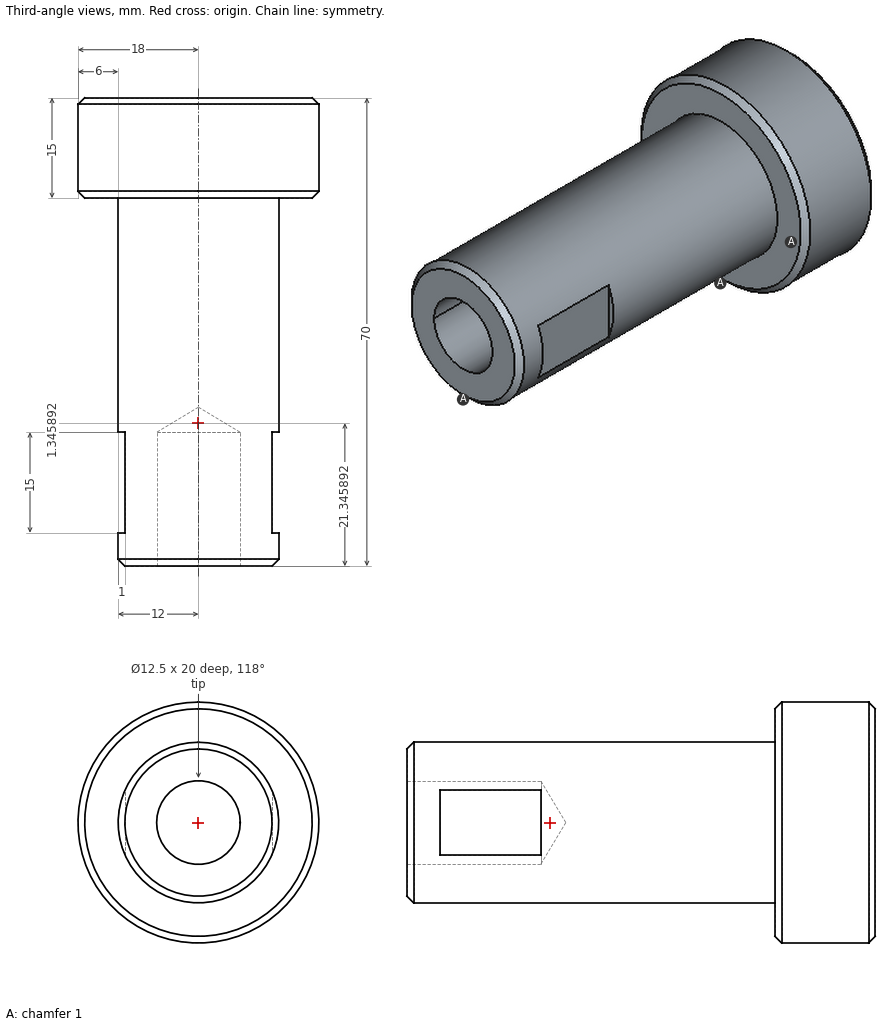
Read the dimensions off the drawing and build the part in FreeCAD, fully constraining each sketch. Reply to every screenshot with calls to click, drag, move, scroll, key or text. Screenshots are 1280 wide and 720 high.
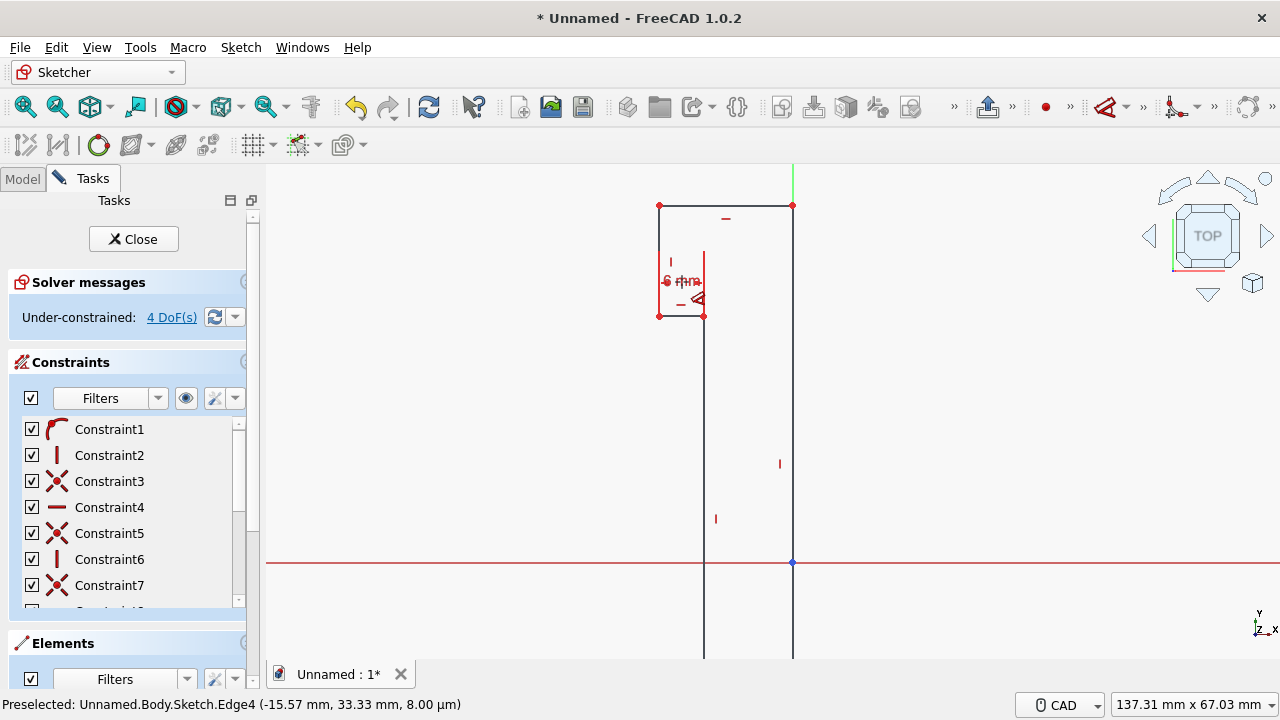
click(793, 567)
click(827, 418)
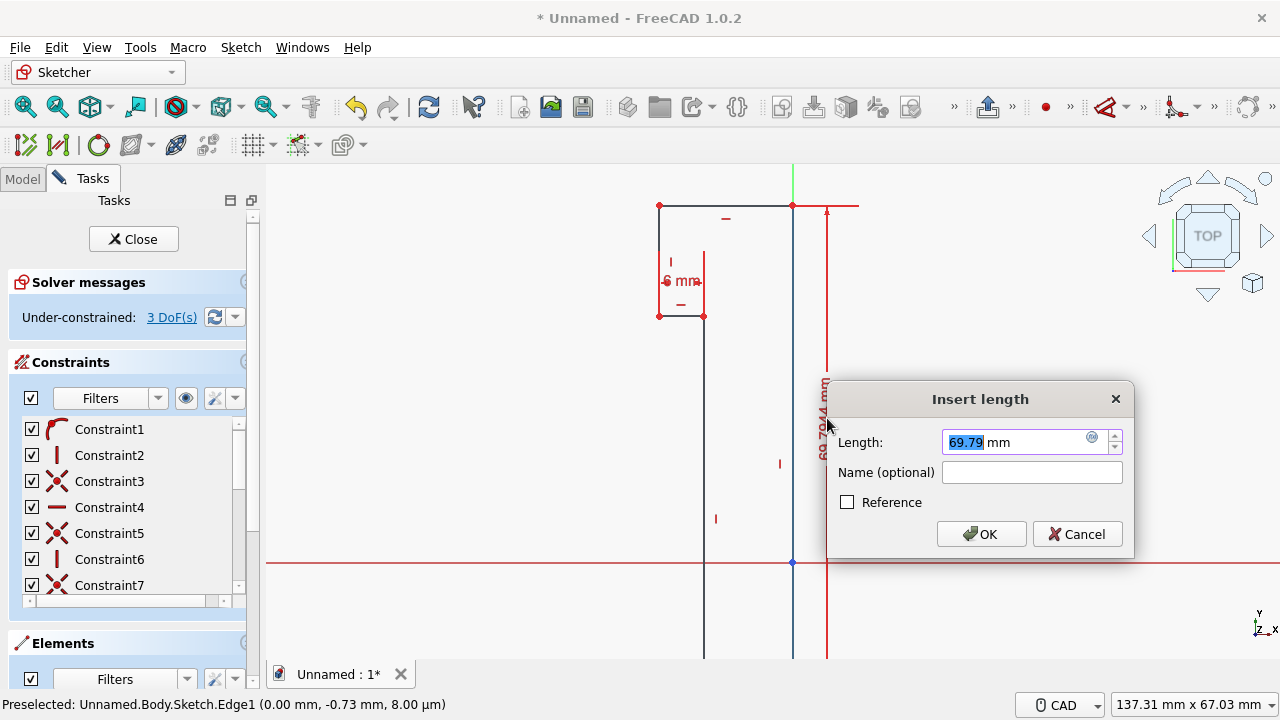
text(70)
key(Return)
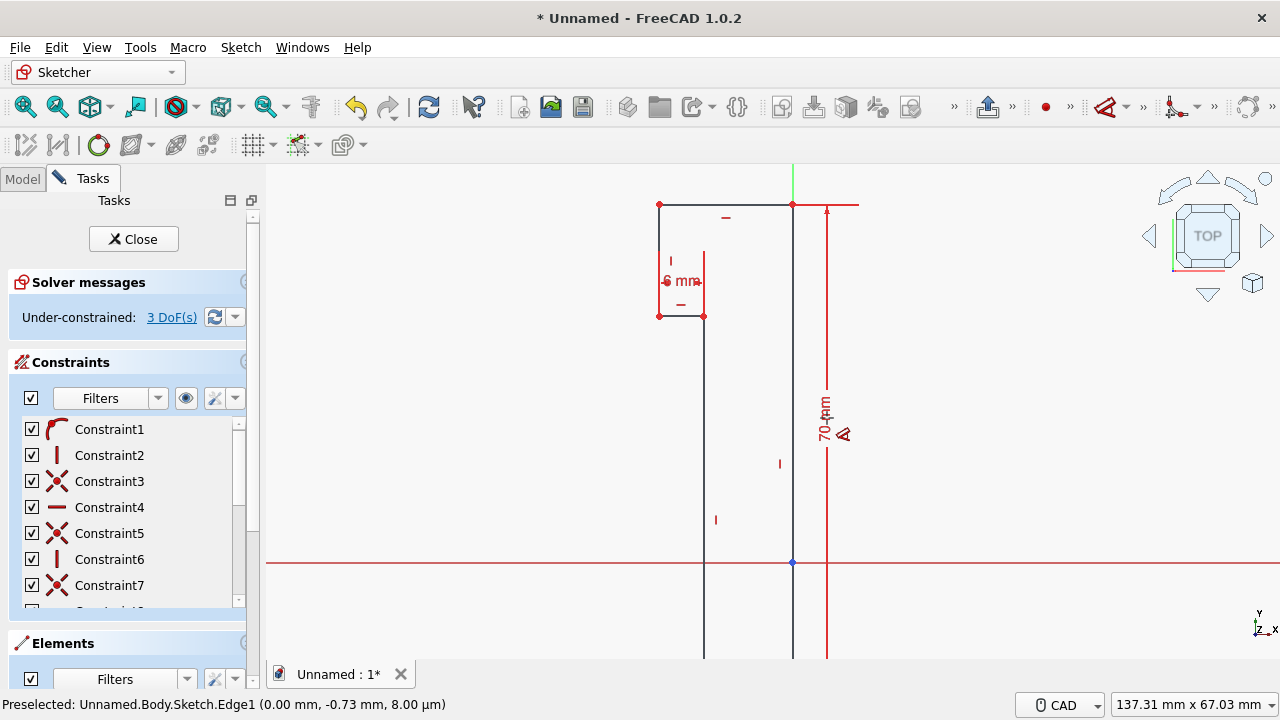
click(753, 205)
click(726, 239)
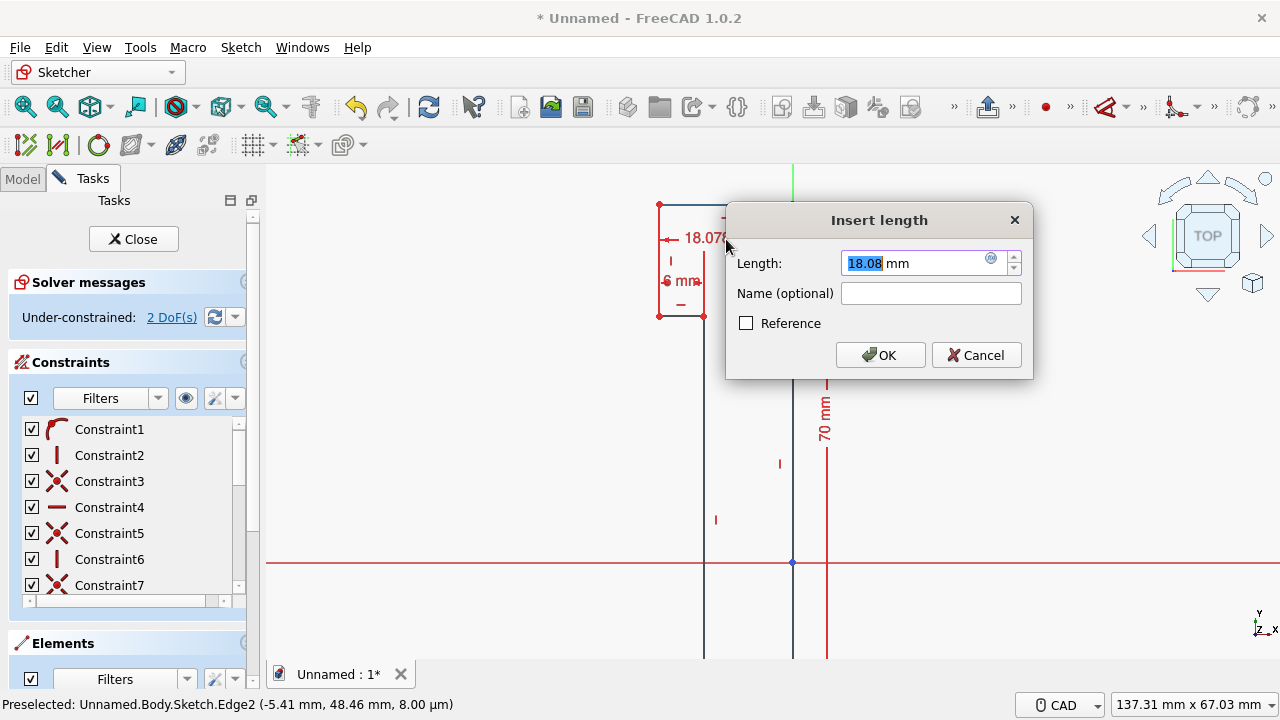
text(18)
key(Return)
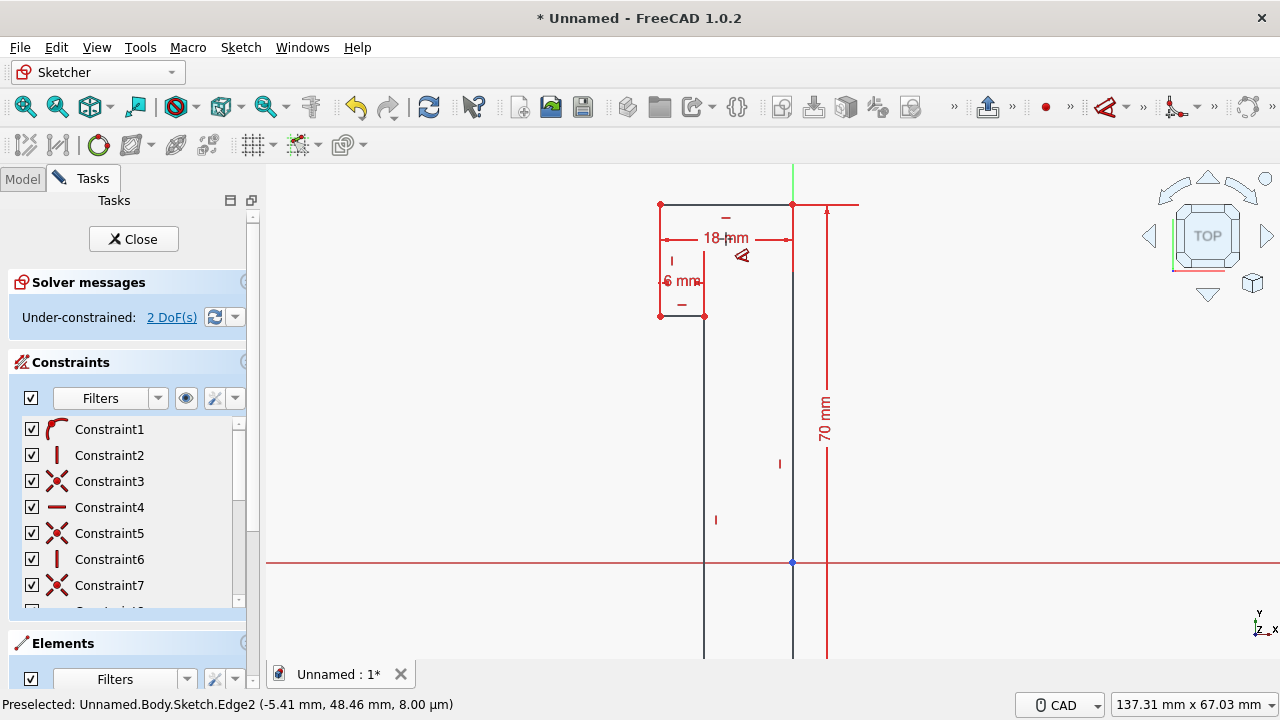
click(660, 238)
click(626, 261)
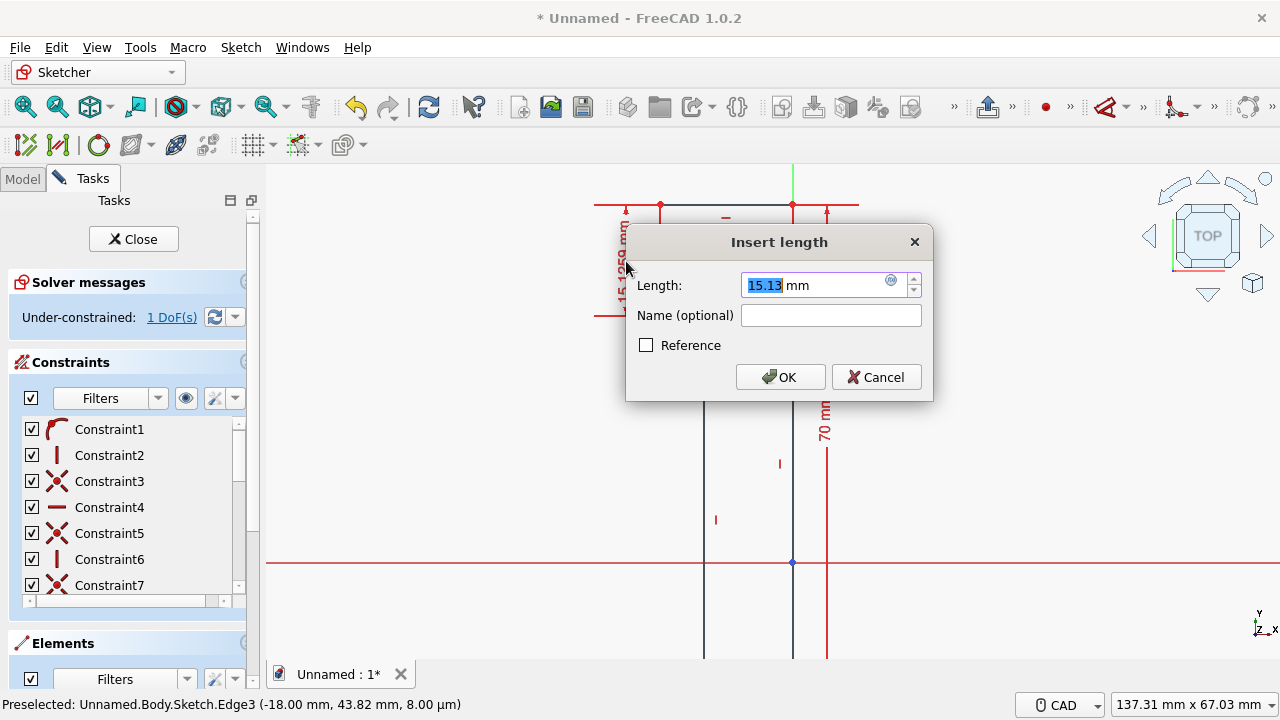
text(15)
key(Return)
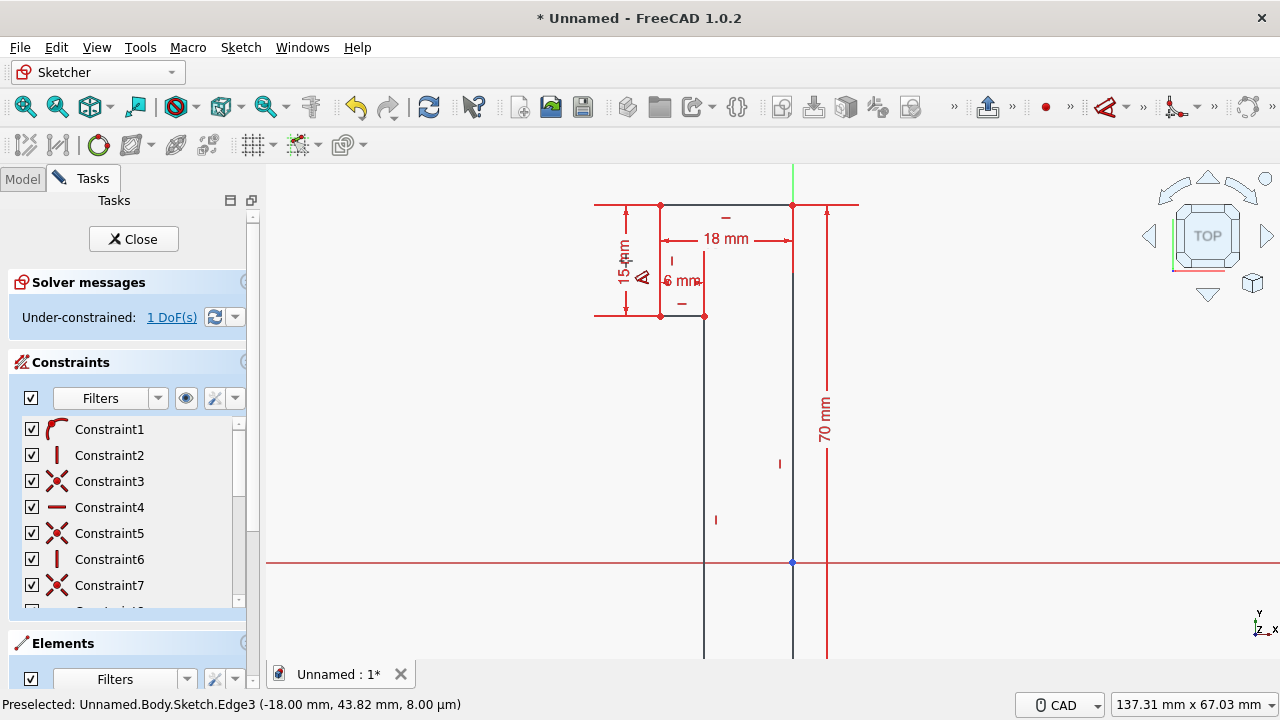
scroll(678, 350, down, 3)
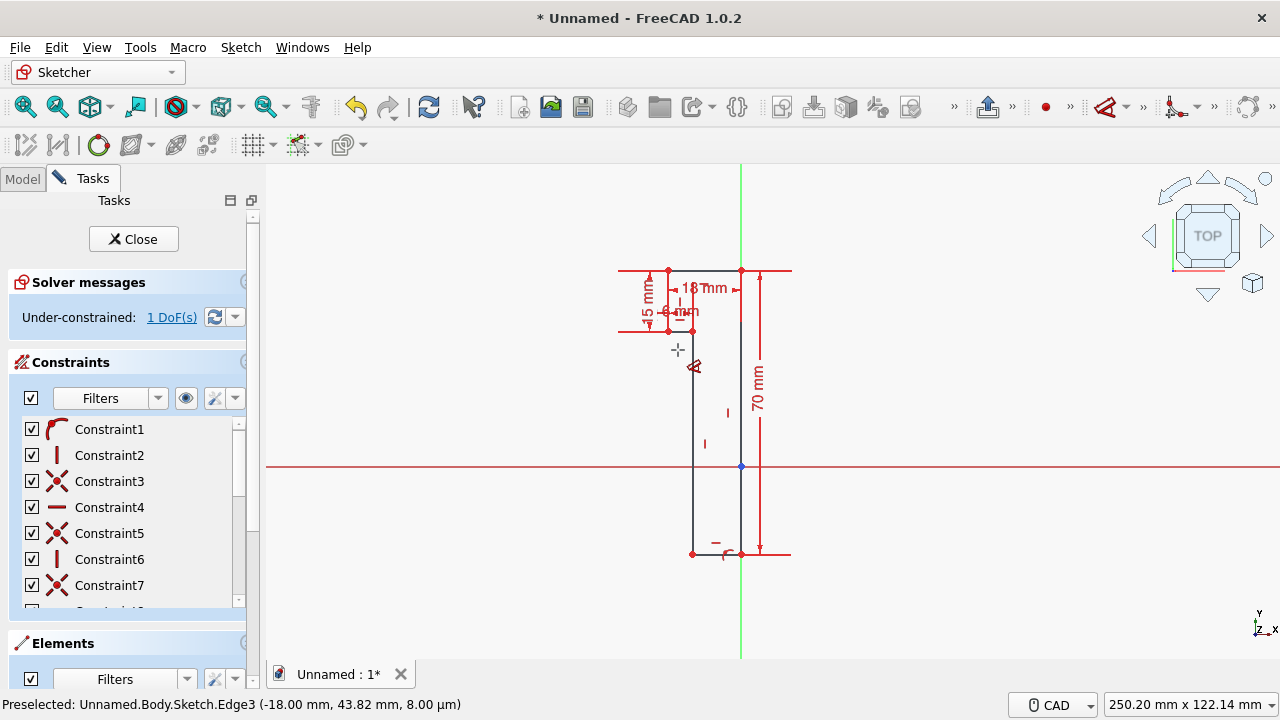
click(741, 555)
click(775, 511)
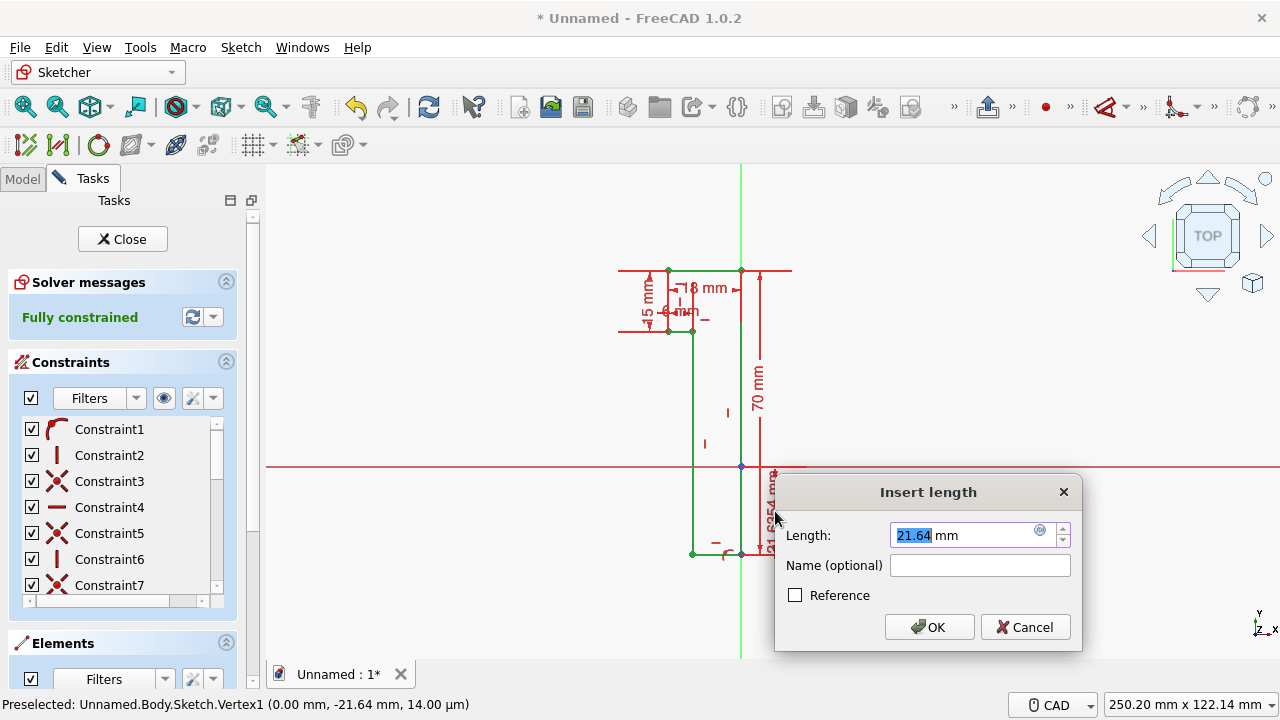
text(21.345892)
key(Return)
key(Escape)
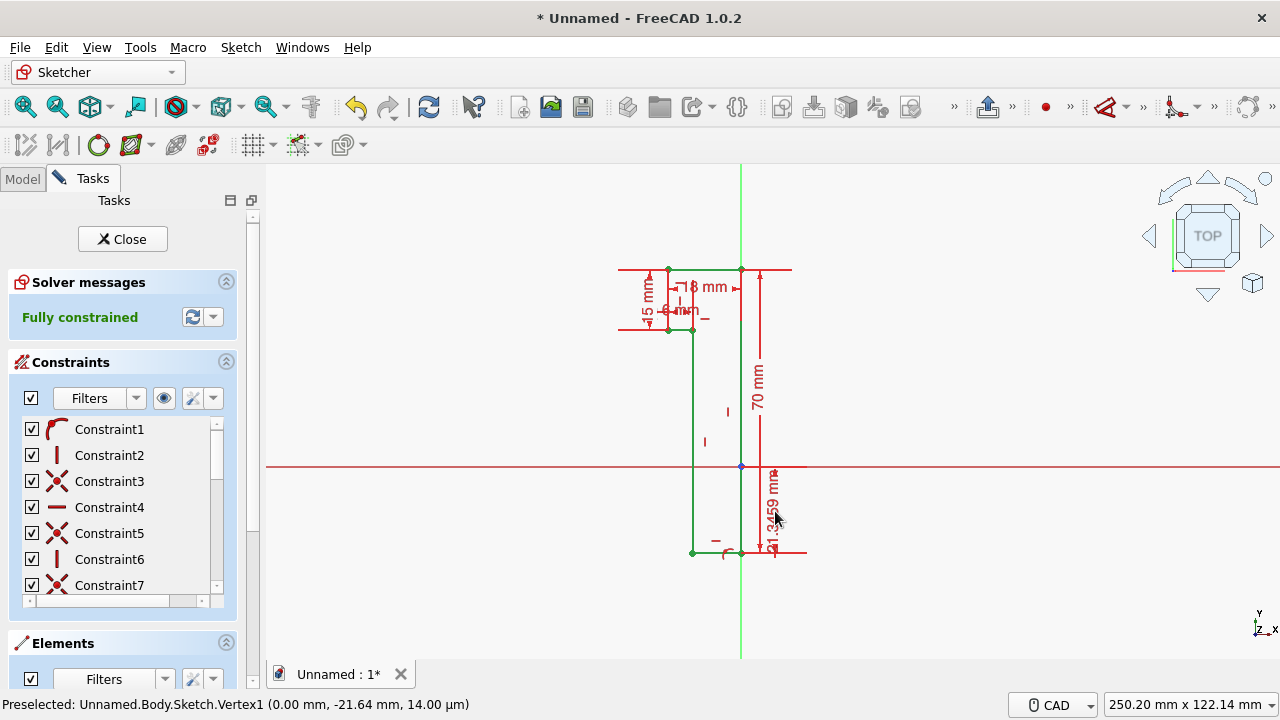
click(123, 239)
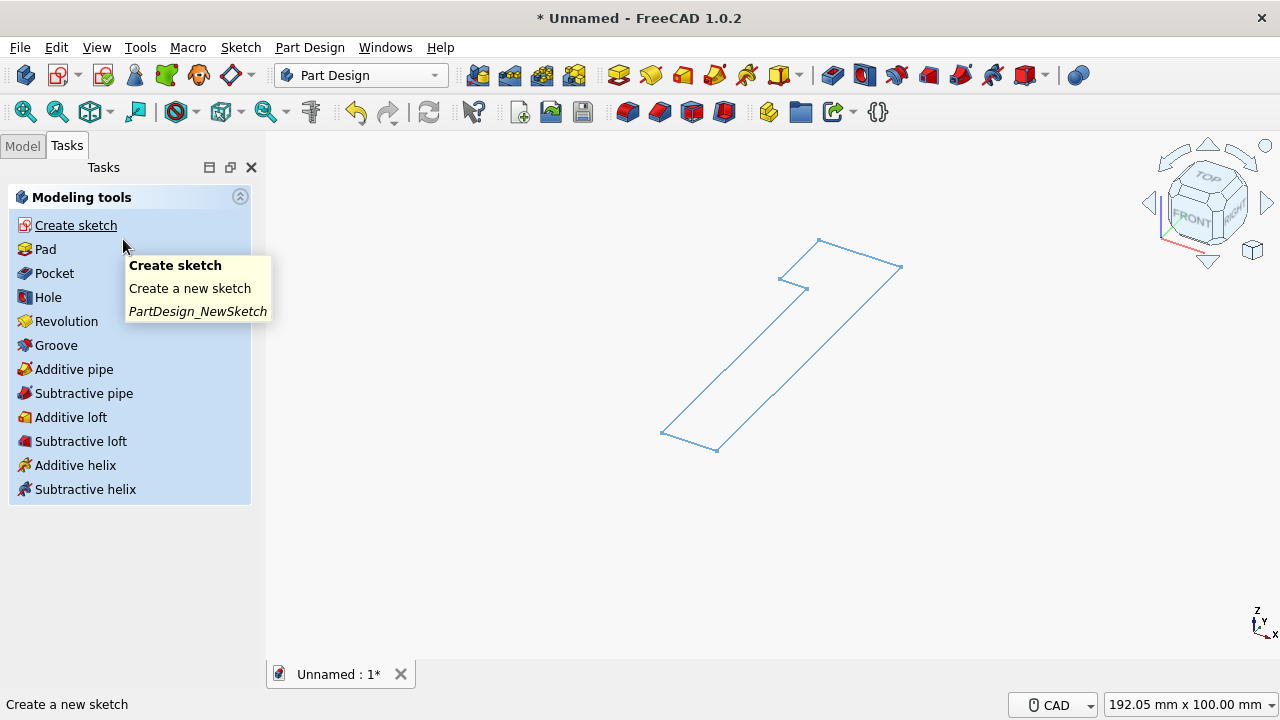
click(652, 76)